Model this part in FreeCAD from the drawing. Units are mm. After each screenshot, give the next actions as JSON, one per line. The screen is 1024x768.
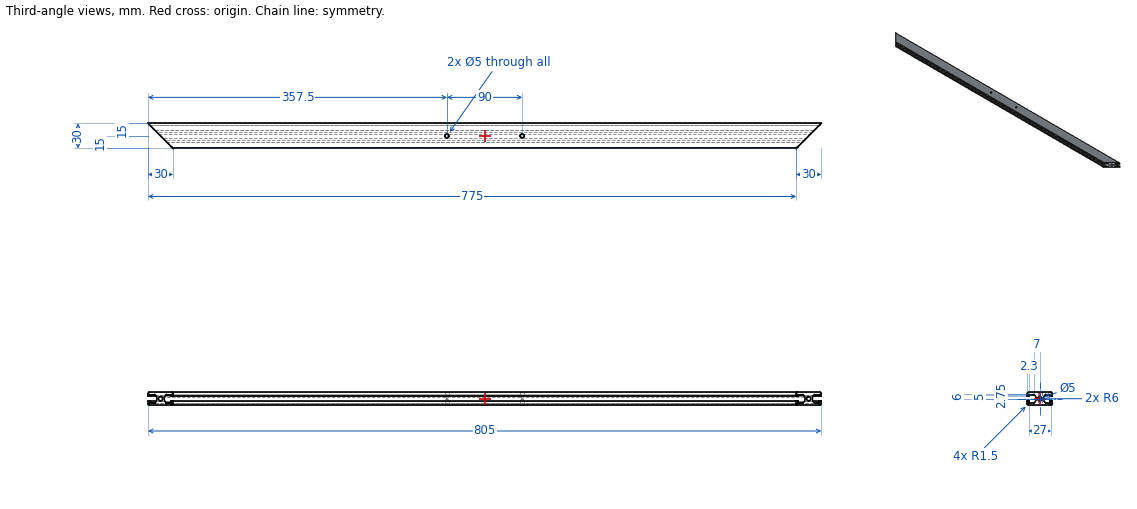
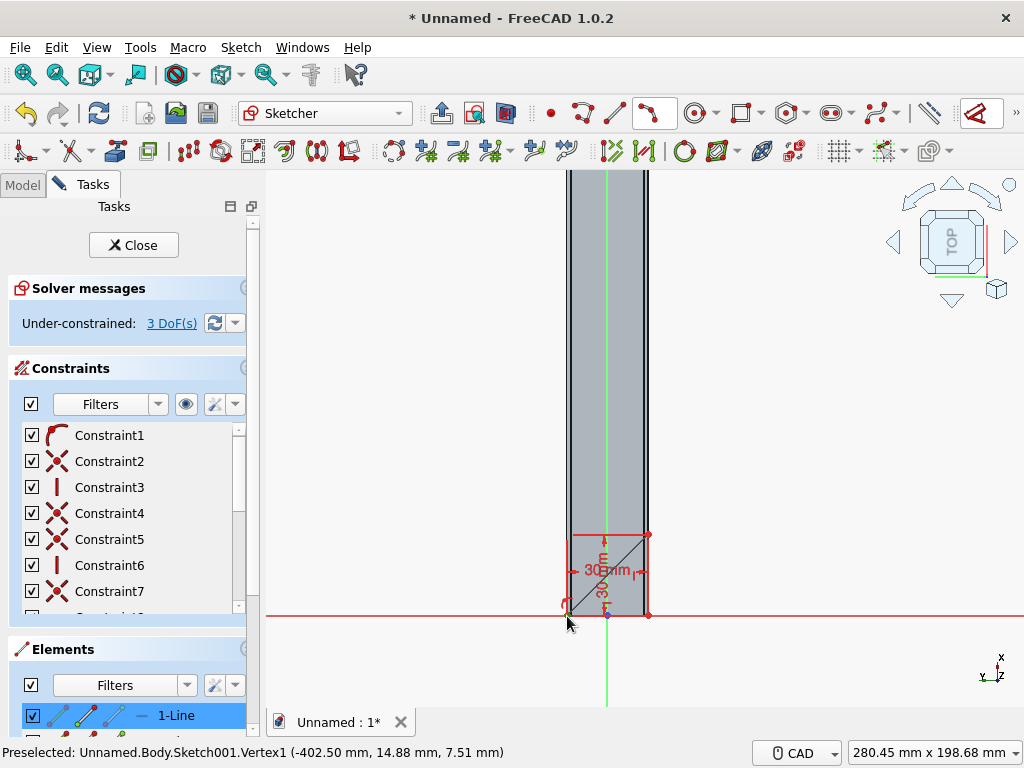
{"action": "key", "text": "l"}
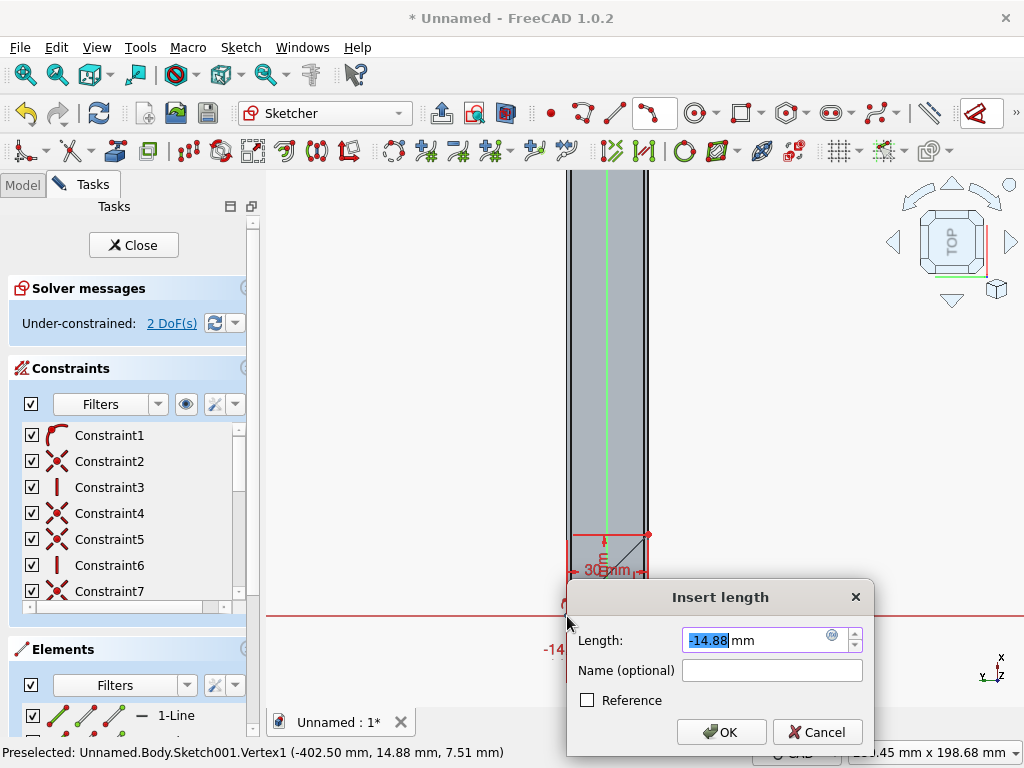
{"action": "type", "text": "-15"}
{"action": "key", "text": "Return"}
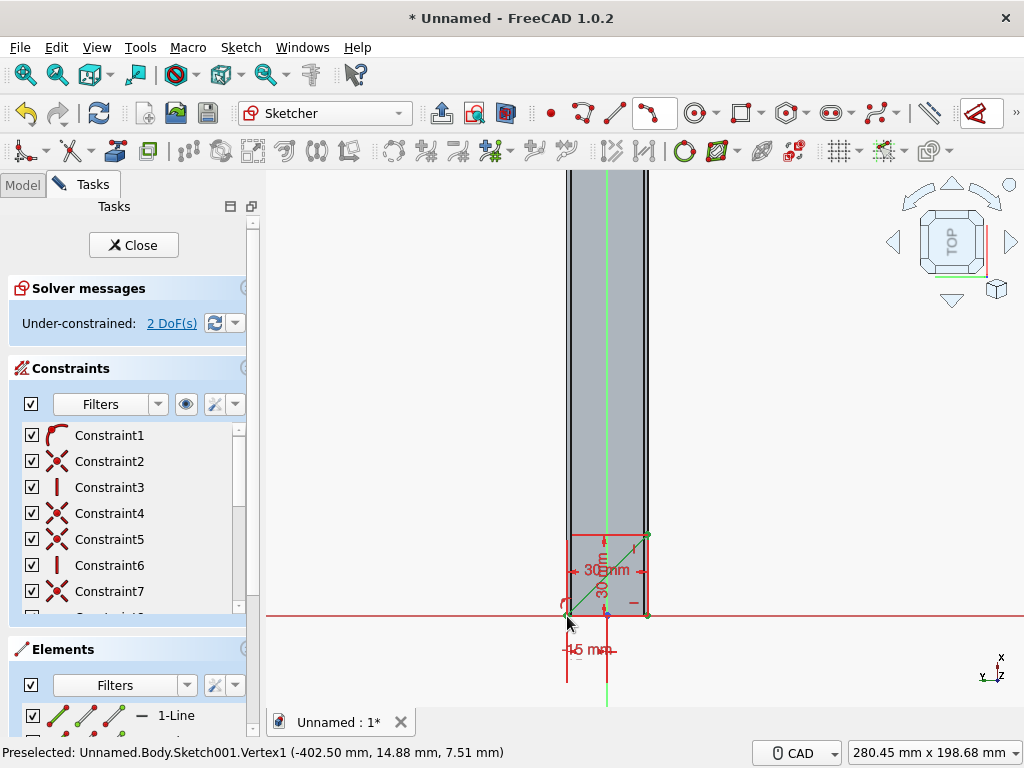
{"action": "scroll", "coordinate": [570, 619], "scroll_direction": "down", "scroll_amount": 9}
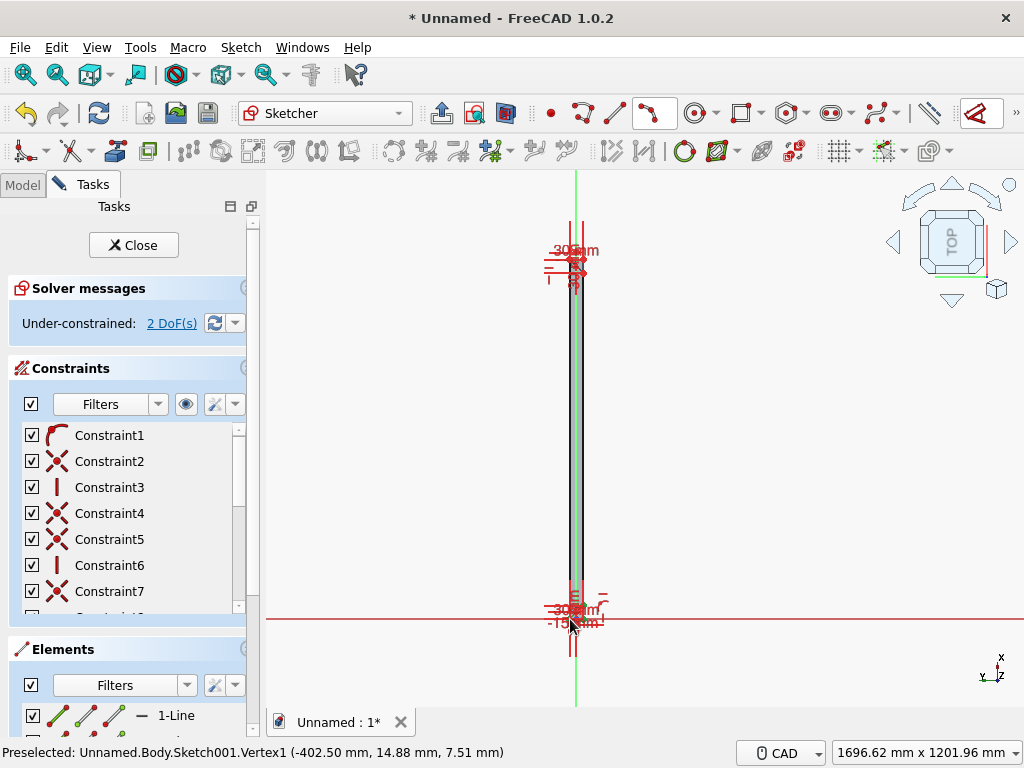
{"action": "scroll", "coordinate": [583, 273], "scroll_direction": "up", "scroll_amount": 9}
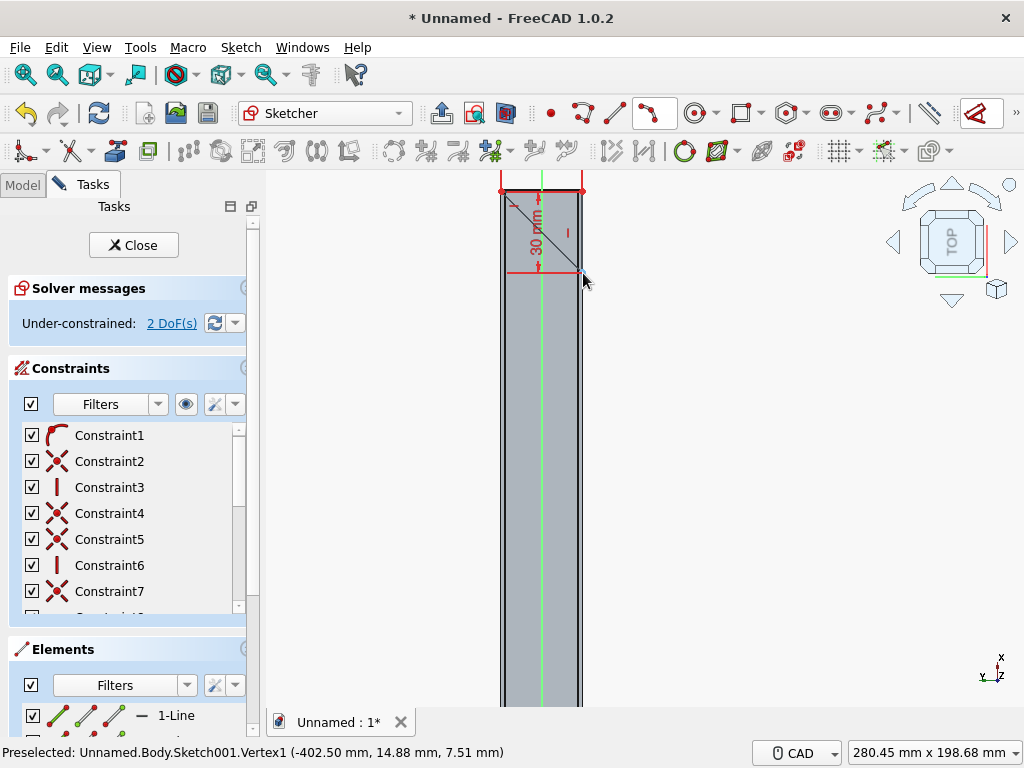
{"action": "left_click", "coordinate": [582, 273]}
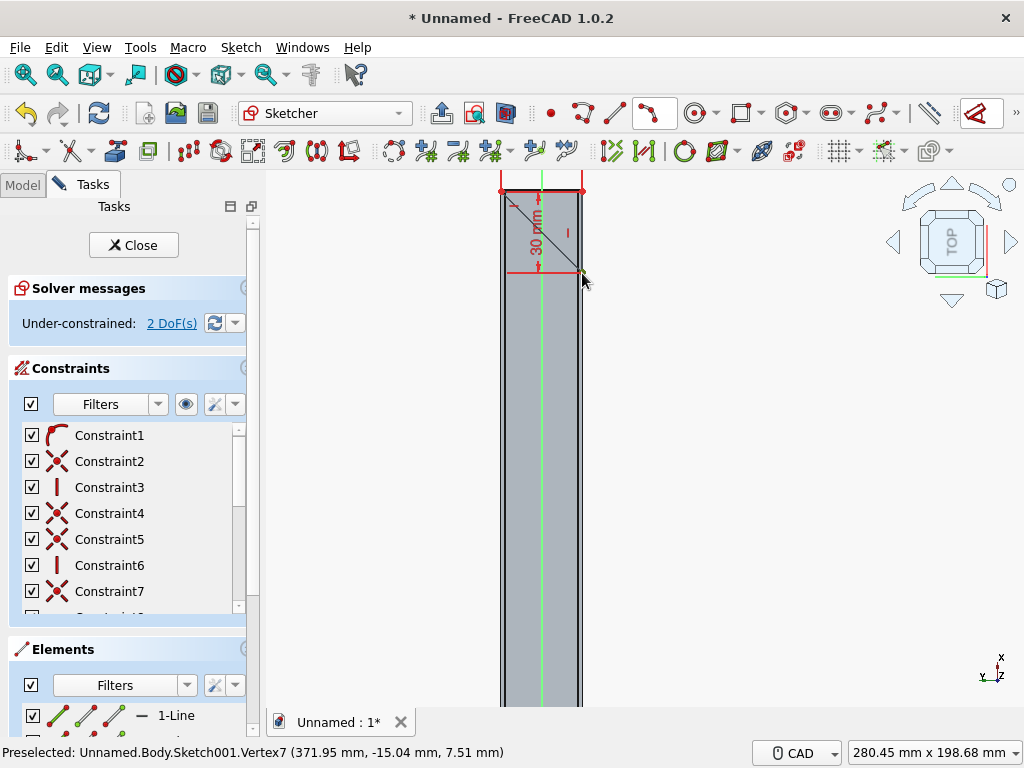
{"action": "key", "text": "l"}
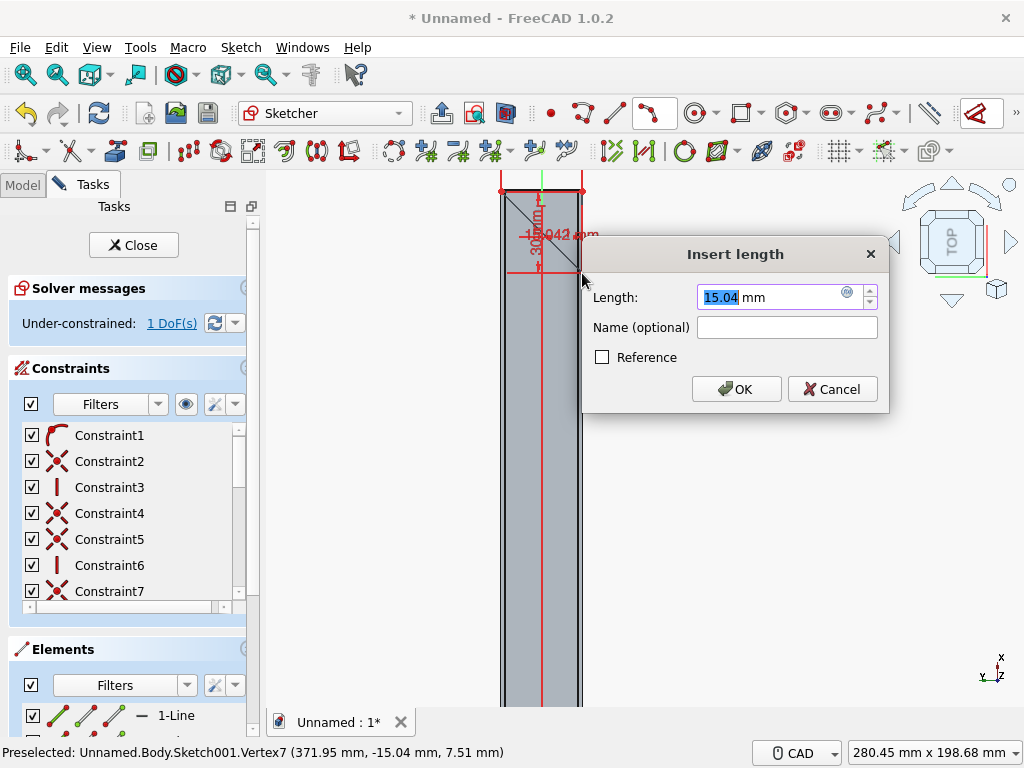
{"action": "type", "text": "15"}
{"action": "key", "text": "Return"}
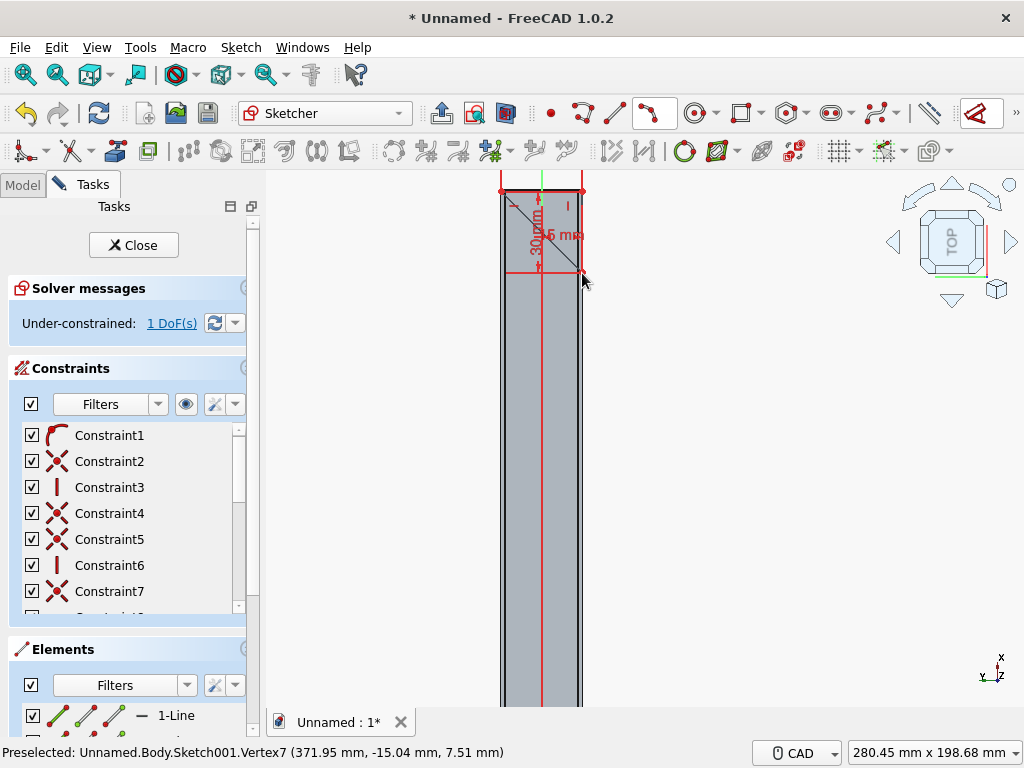
{"action": "scroll", "coordinate": [583, 272], "scroll_direction": "down", "scroll_amount": 9}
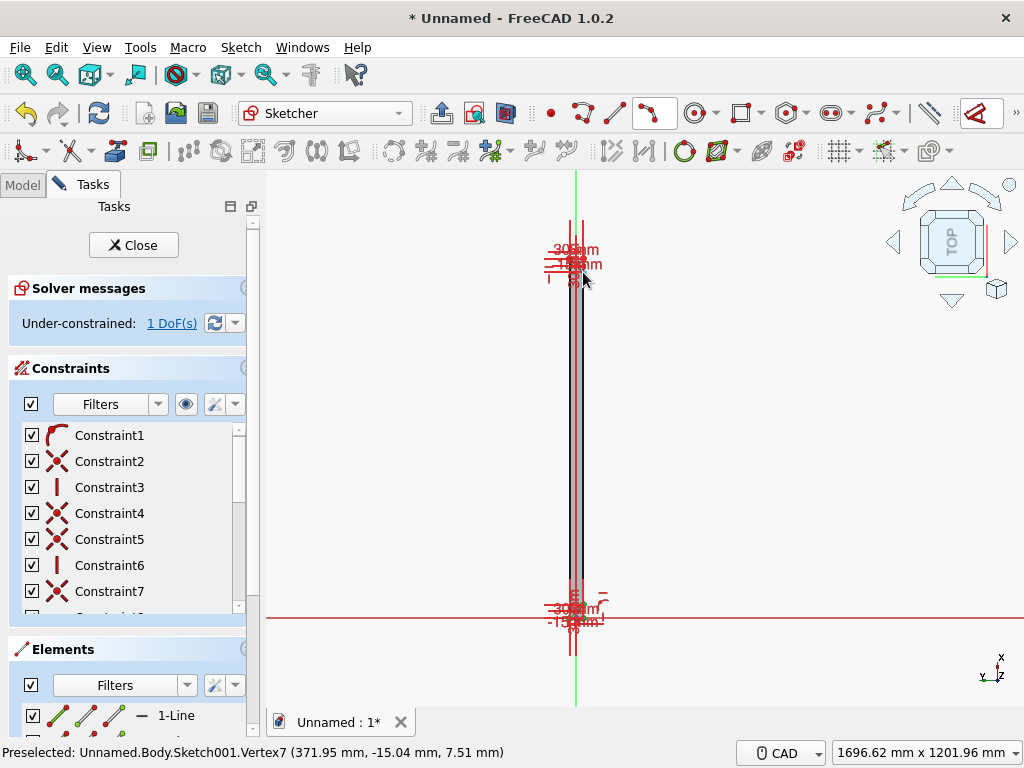
{"action": "left_click", "coordinate": [583, 272]}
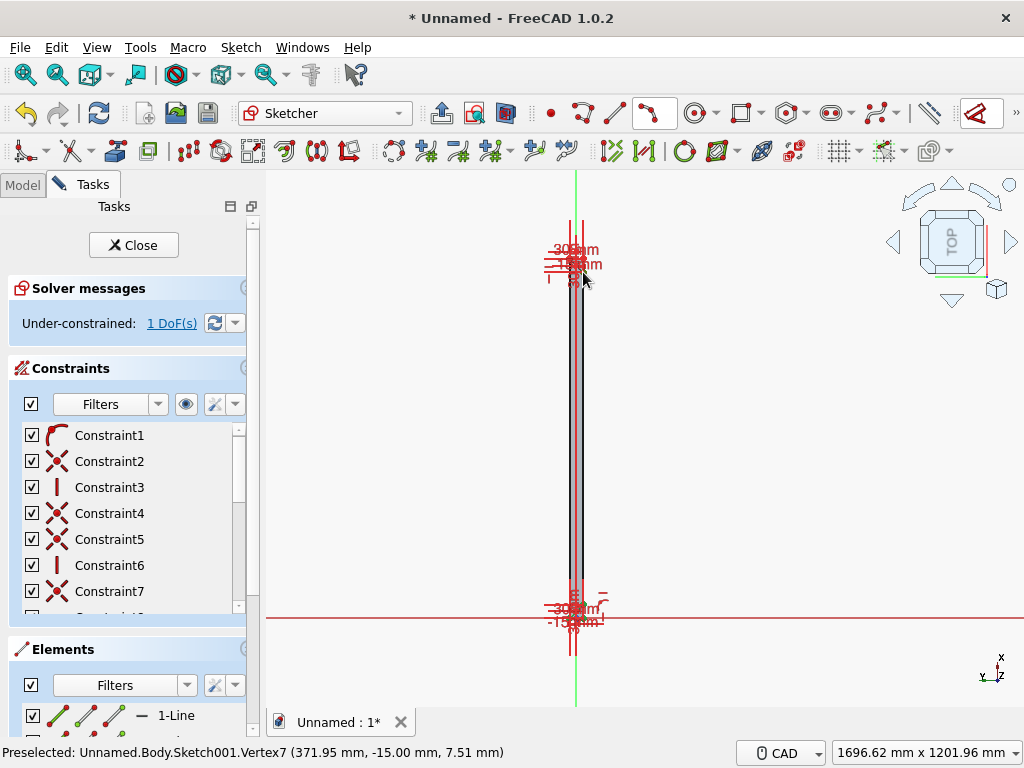
{"action": "key", "text": "i"}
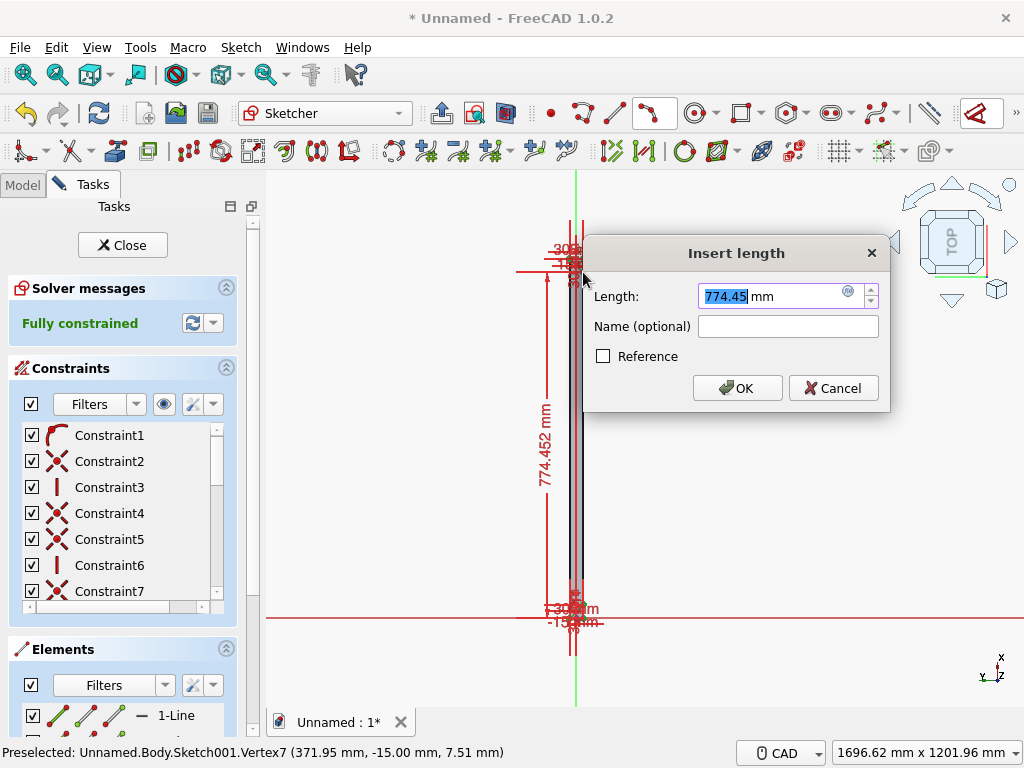
{"action": "type", "text": "775"}
{"action": "key", "text": "Return"}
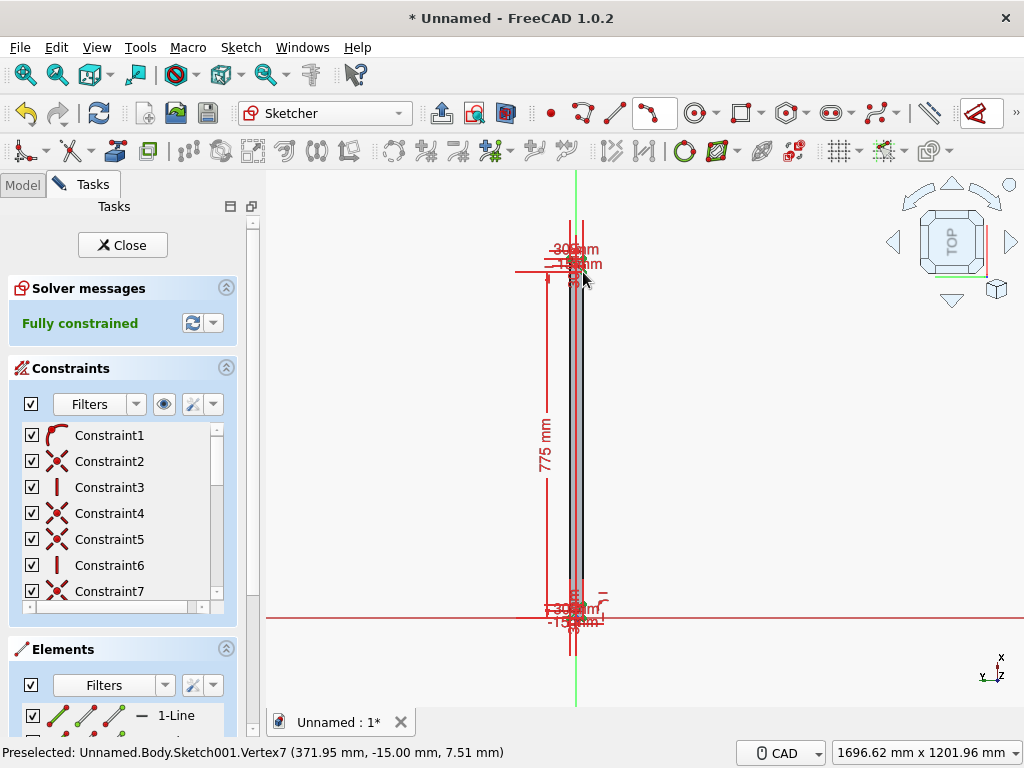
{"action": "left_click", "coordinate": [123, 245]}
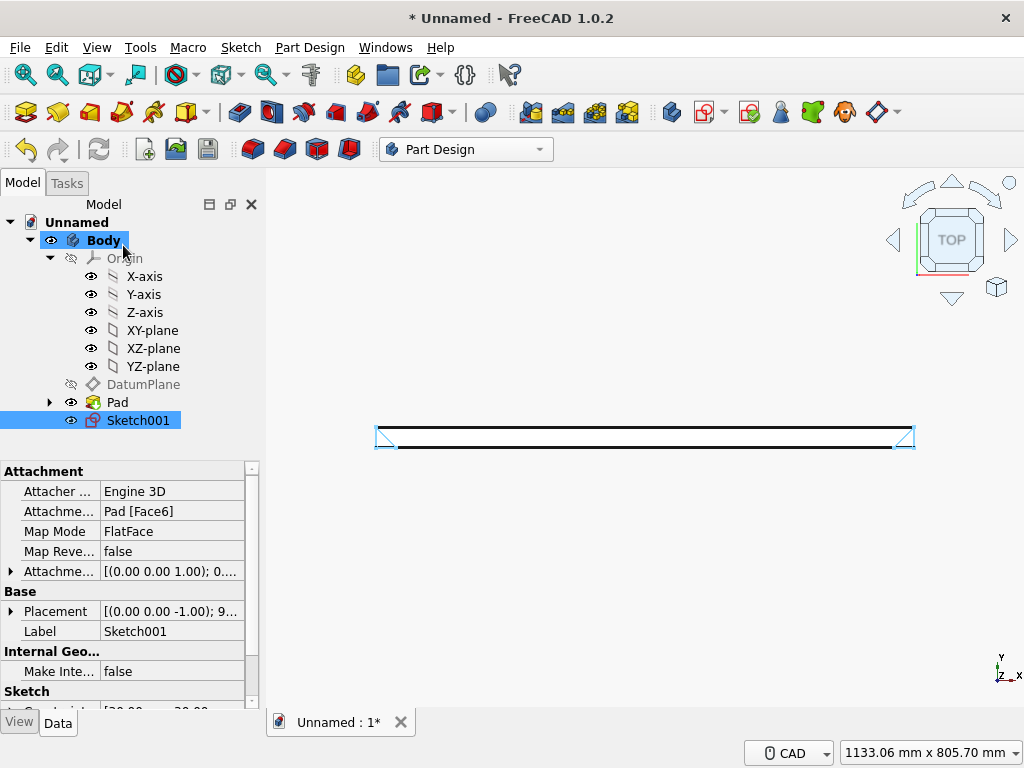
{"action": "left_click", "coordinate": [240, 112]}